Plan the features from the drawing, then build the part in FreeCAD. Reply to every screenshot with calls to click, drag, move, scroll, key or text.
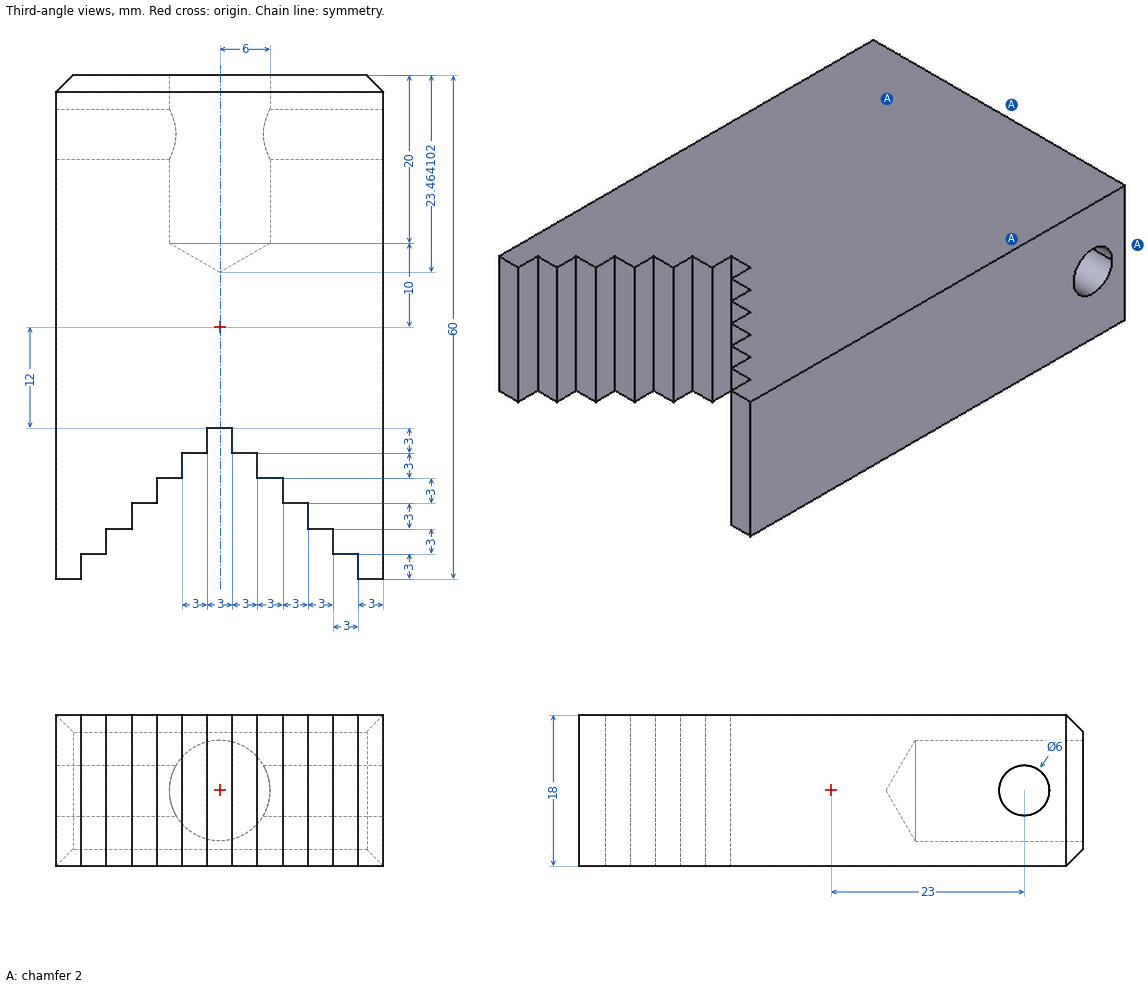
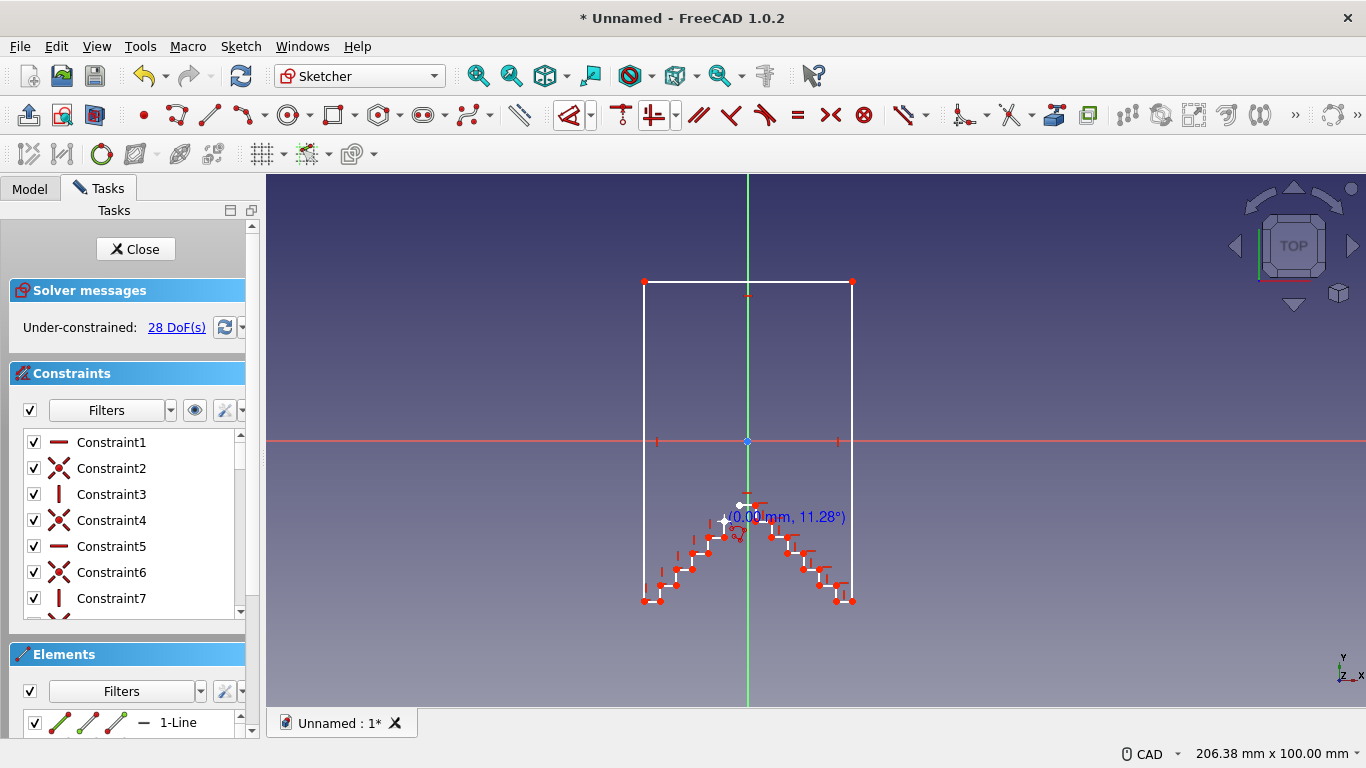
scroll(740, 521, up, 4)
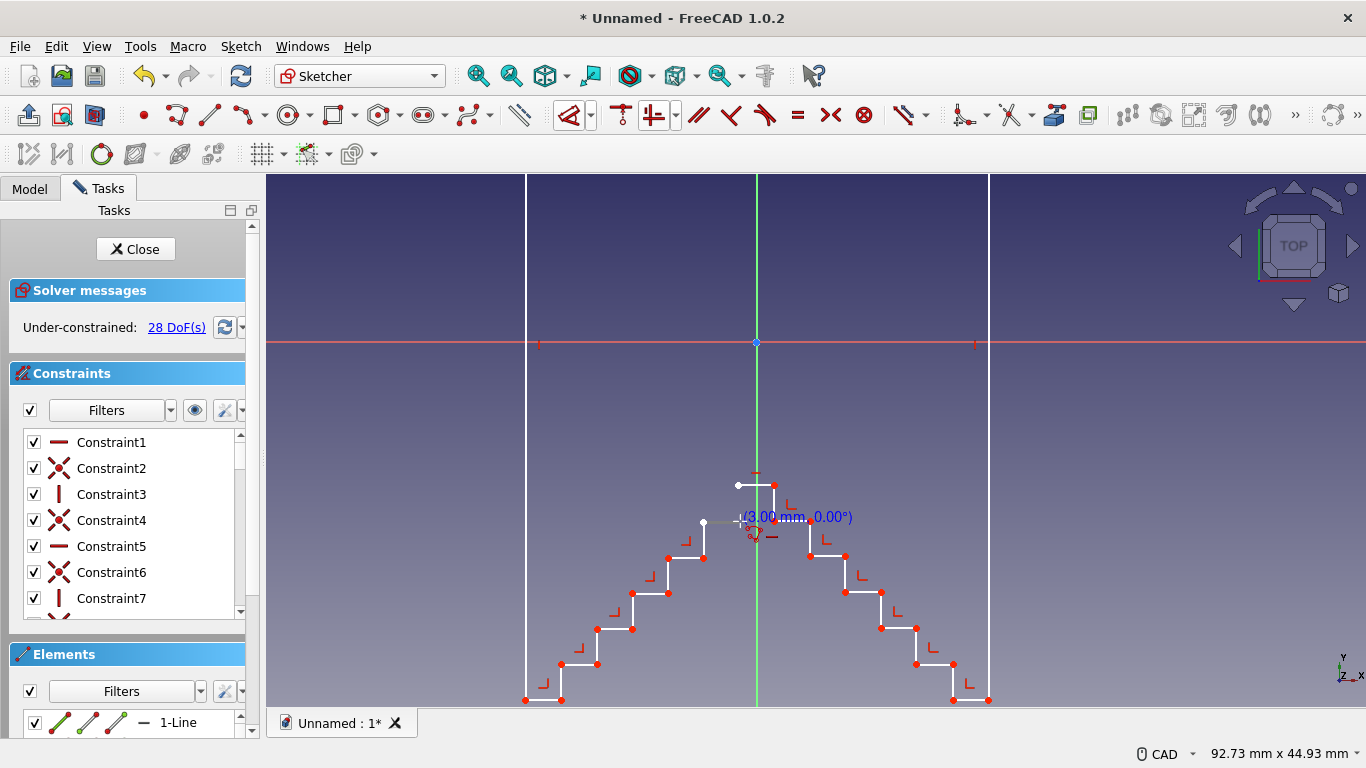
click(739, 520)
click(738, 485)
key(Escape)
key(Escape)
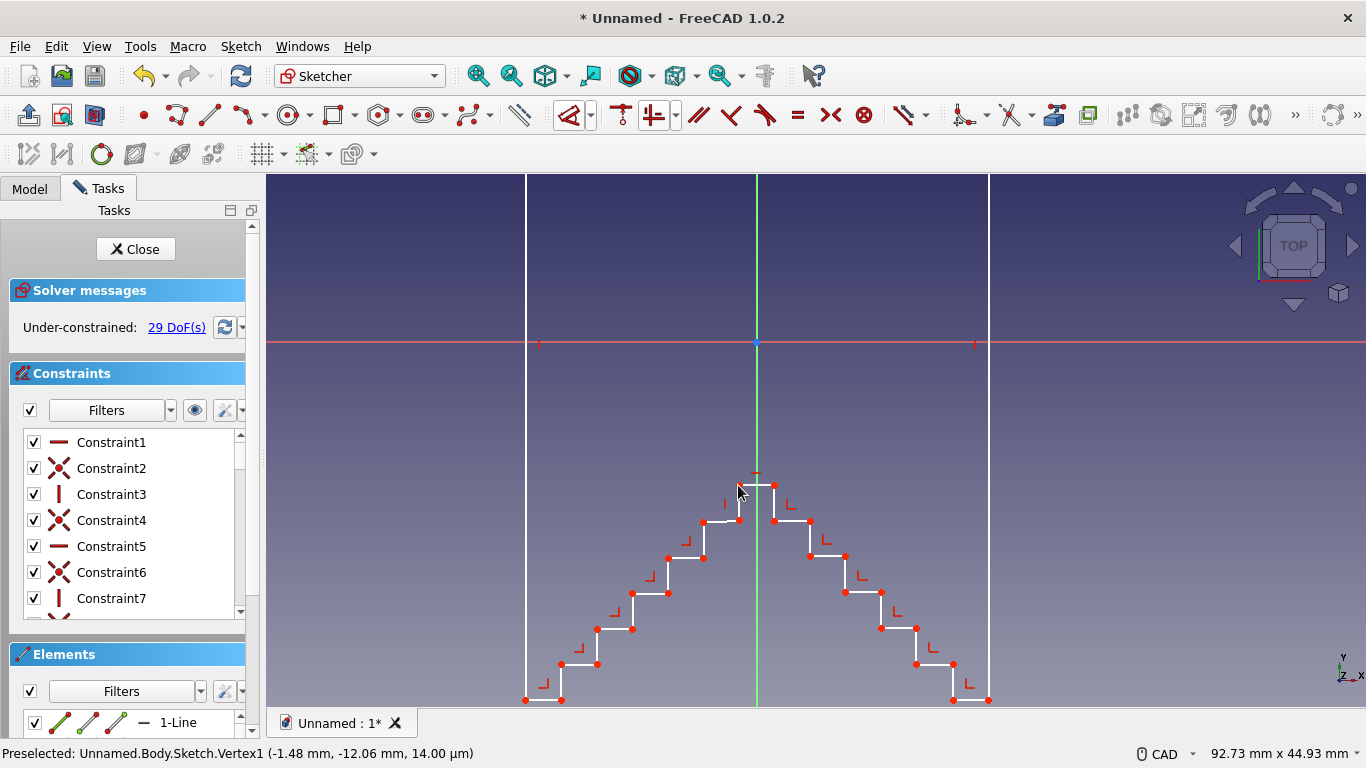
scroll(714, 522, up, 2)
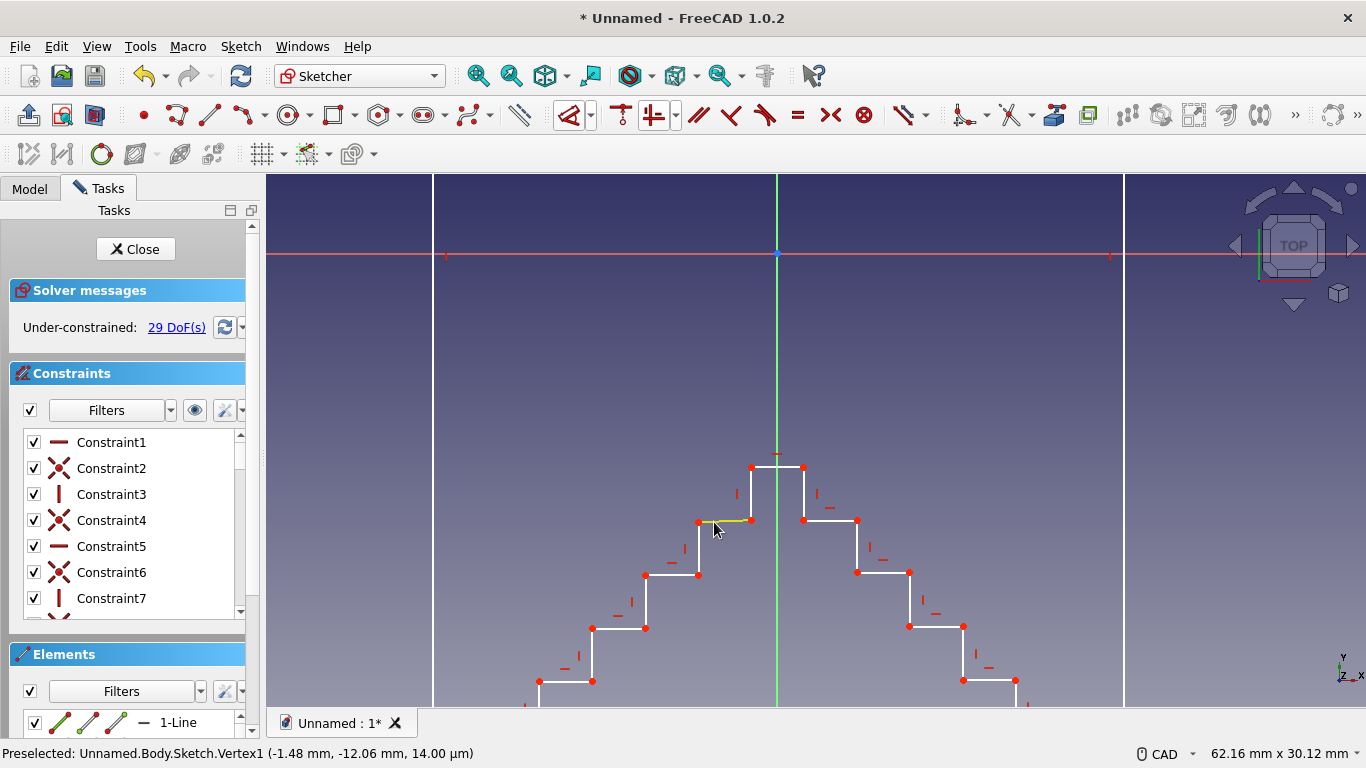
click(714, 522)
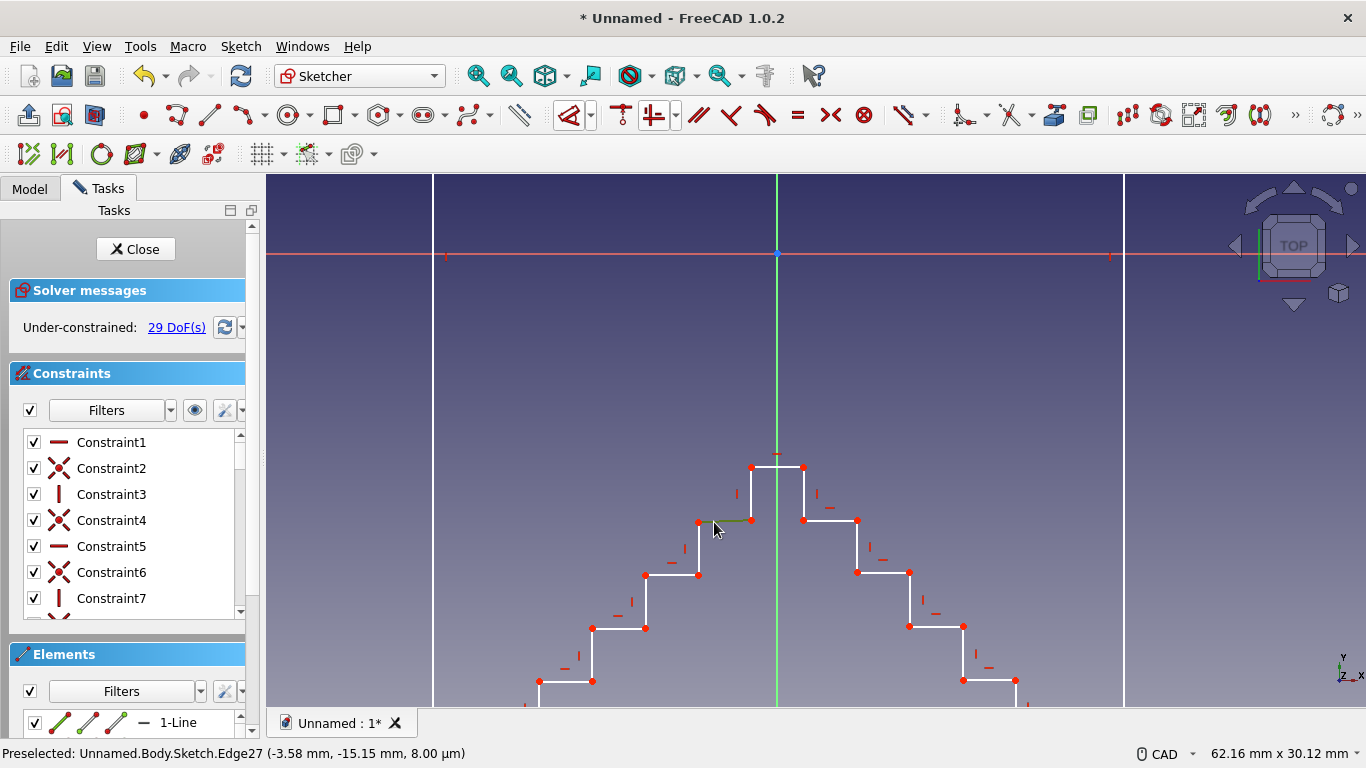
click(676, 116)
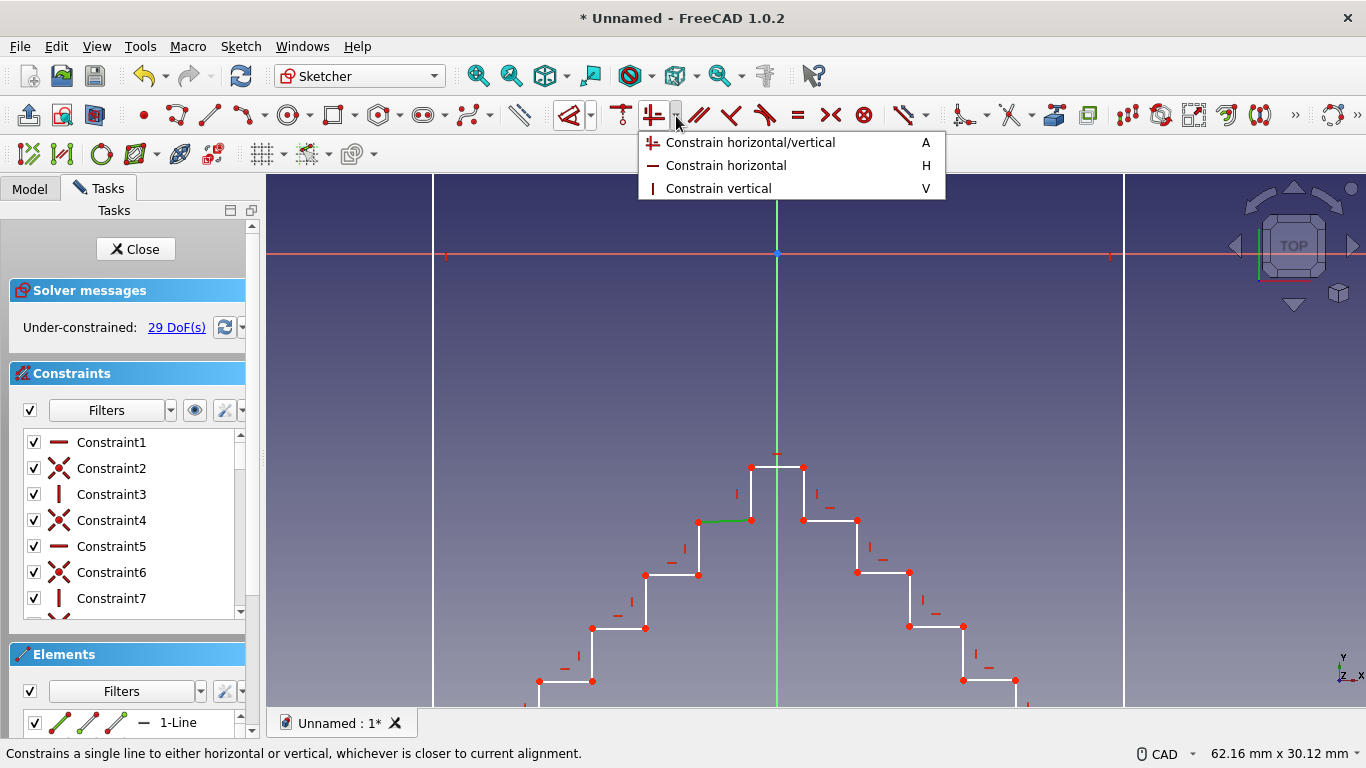
click(792, 166)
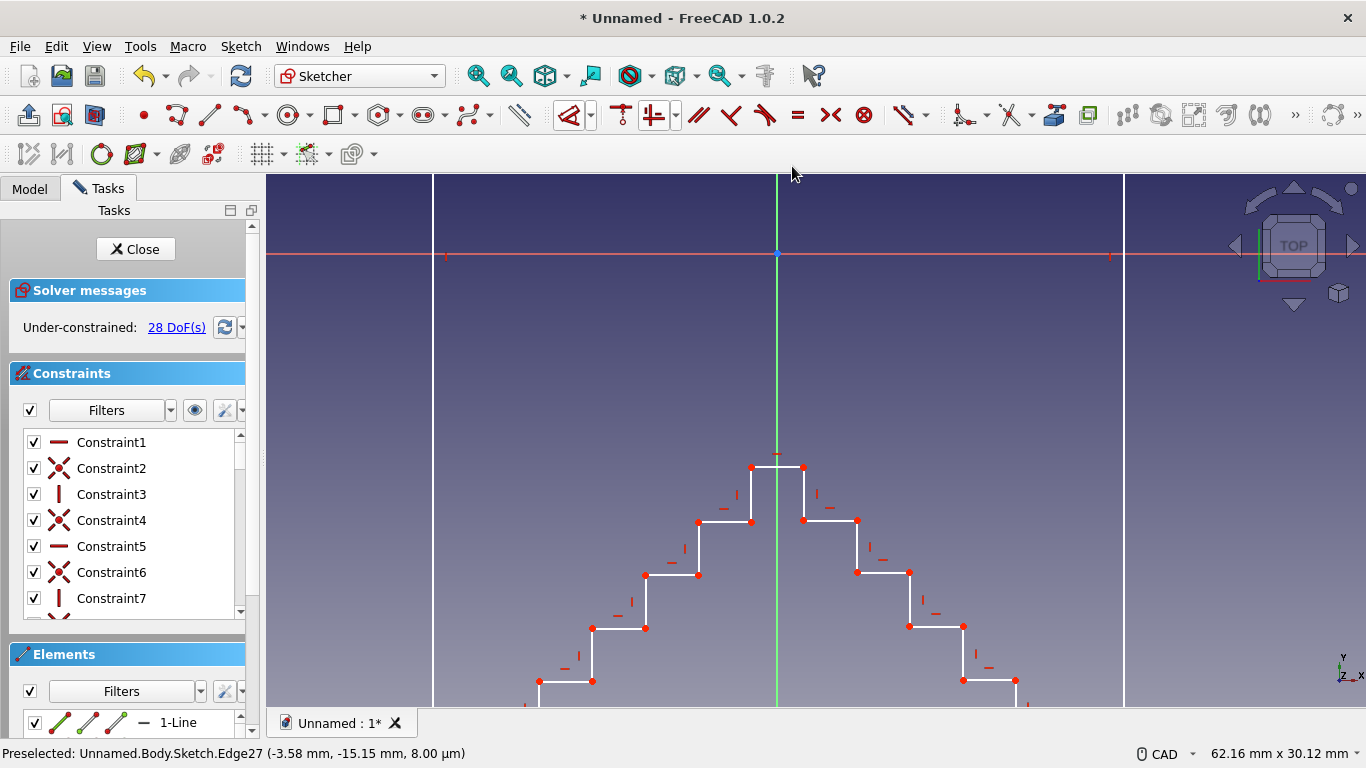
scroll(735, 521, down, 6)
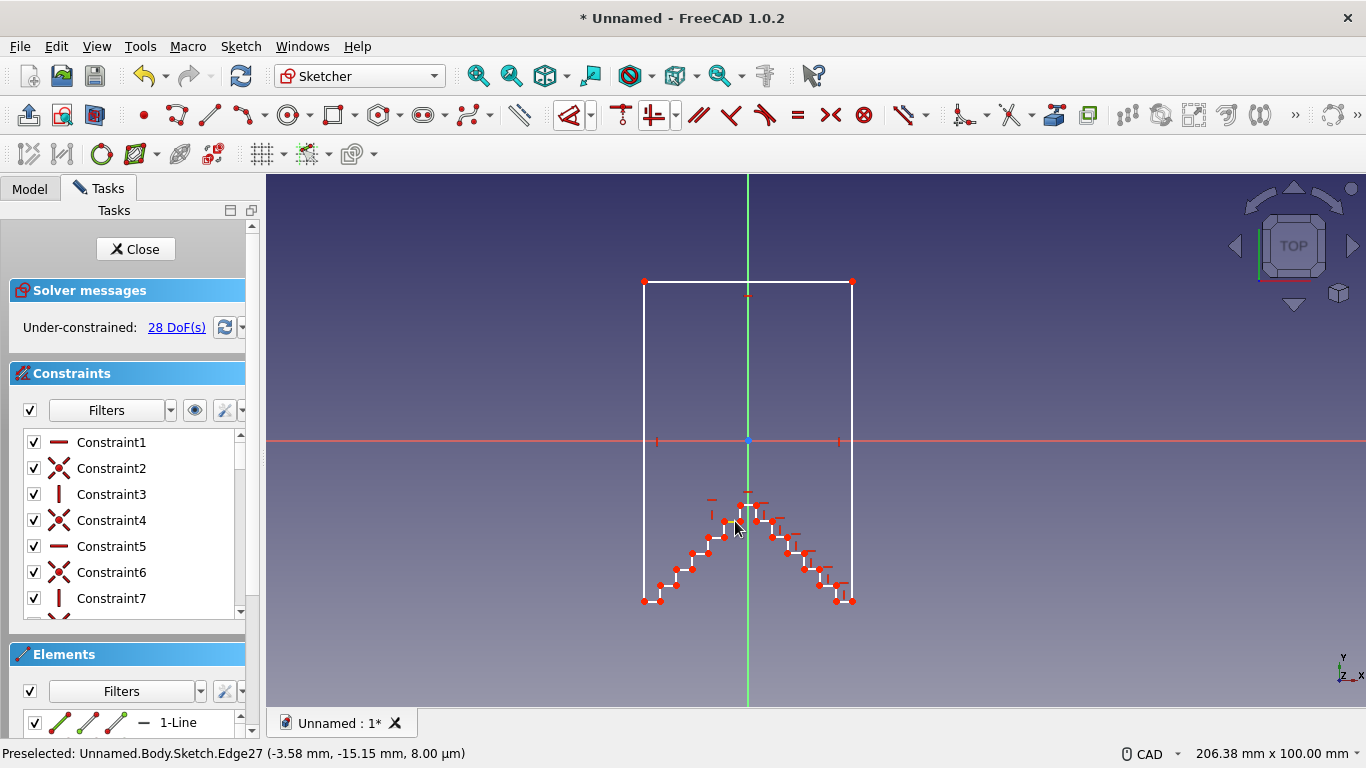
click(852, 602)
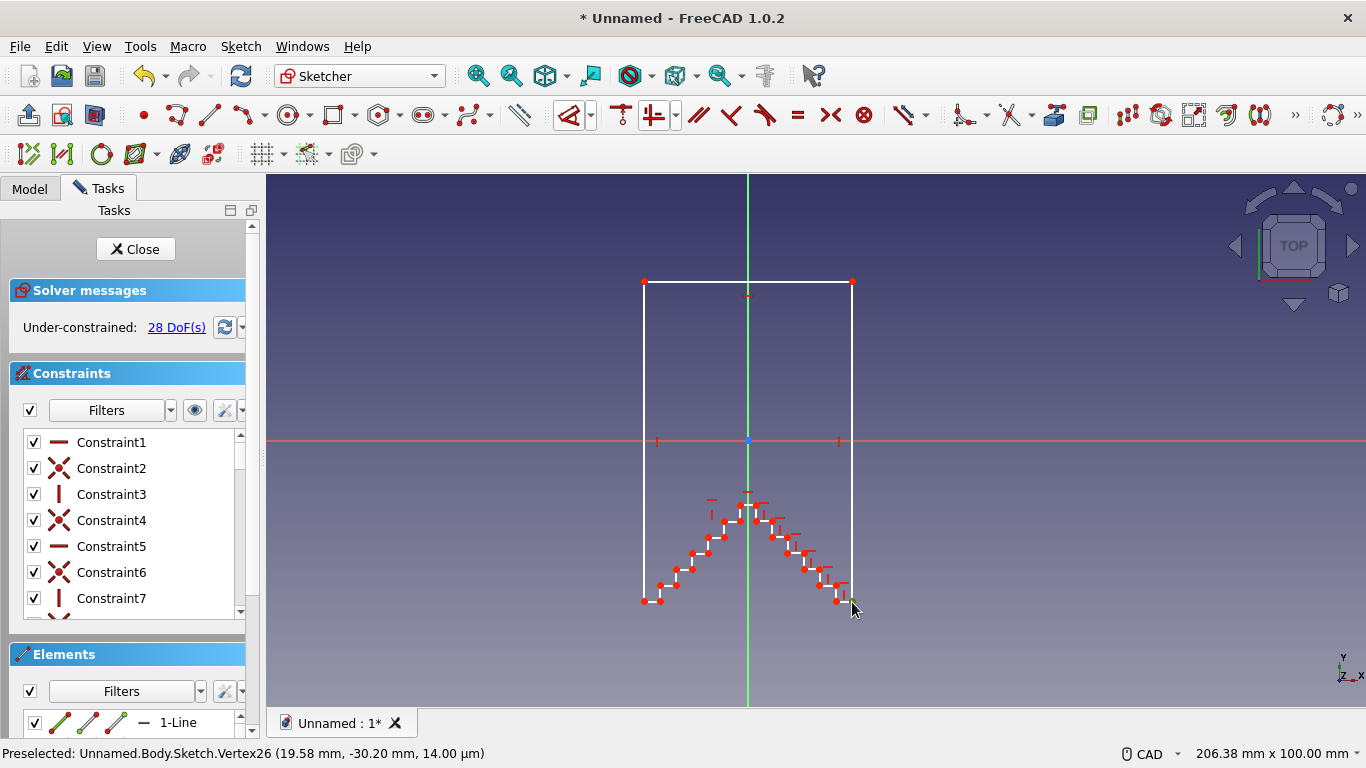
click(644, 602)